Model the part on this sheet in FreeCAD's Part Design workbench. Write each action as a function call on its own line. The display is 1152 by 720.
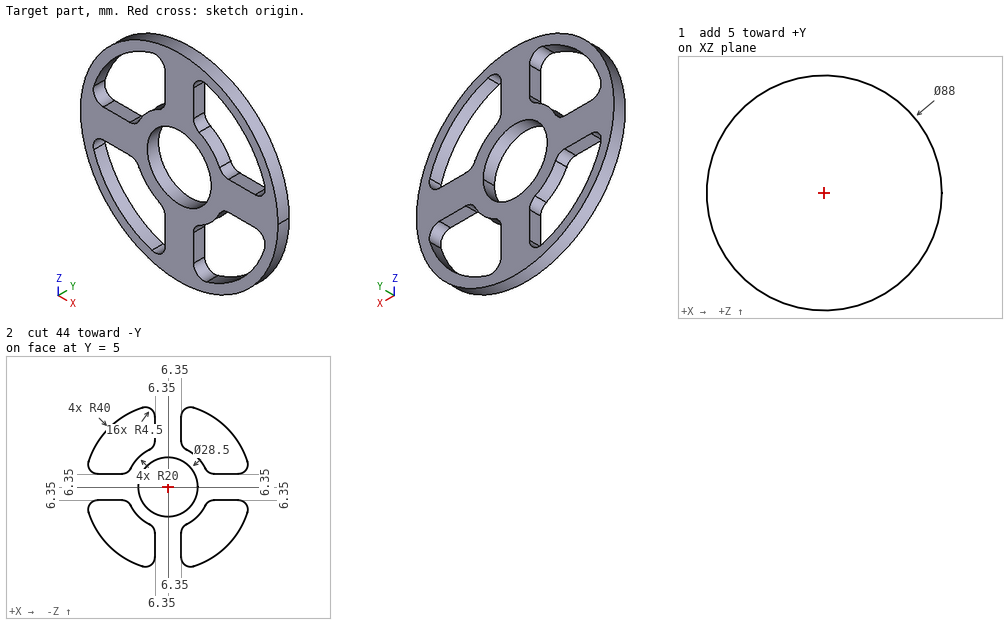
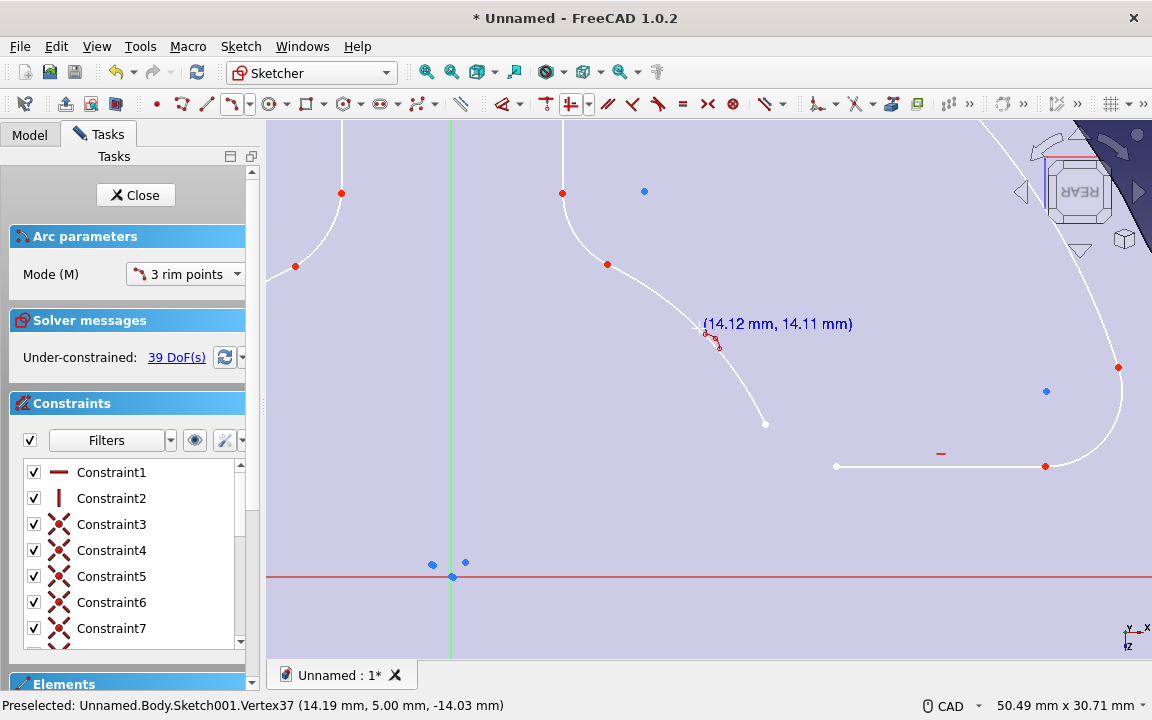
scroll(702, 328, down, 7)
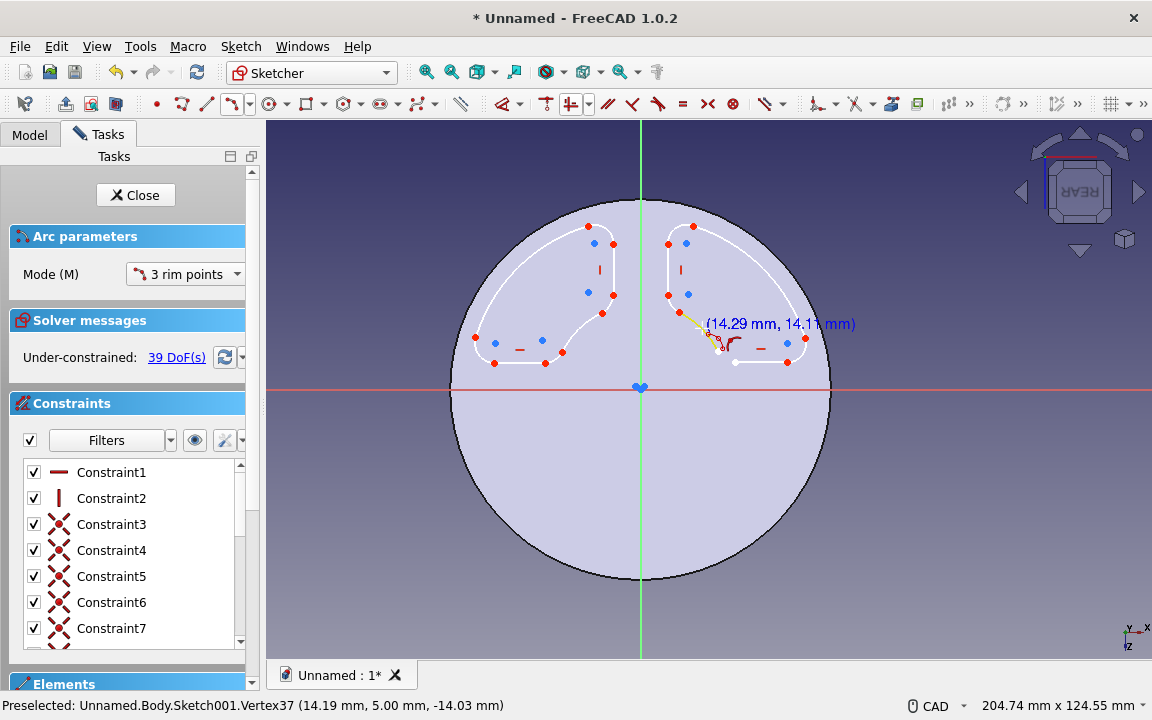
click(718, 352)
click(736, 362)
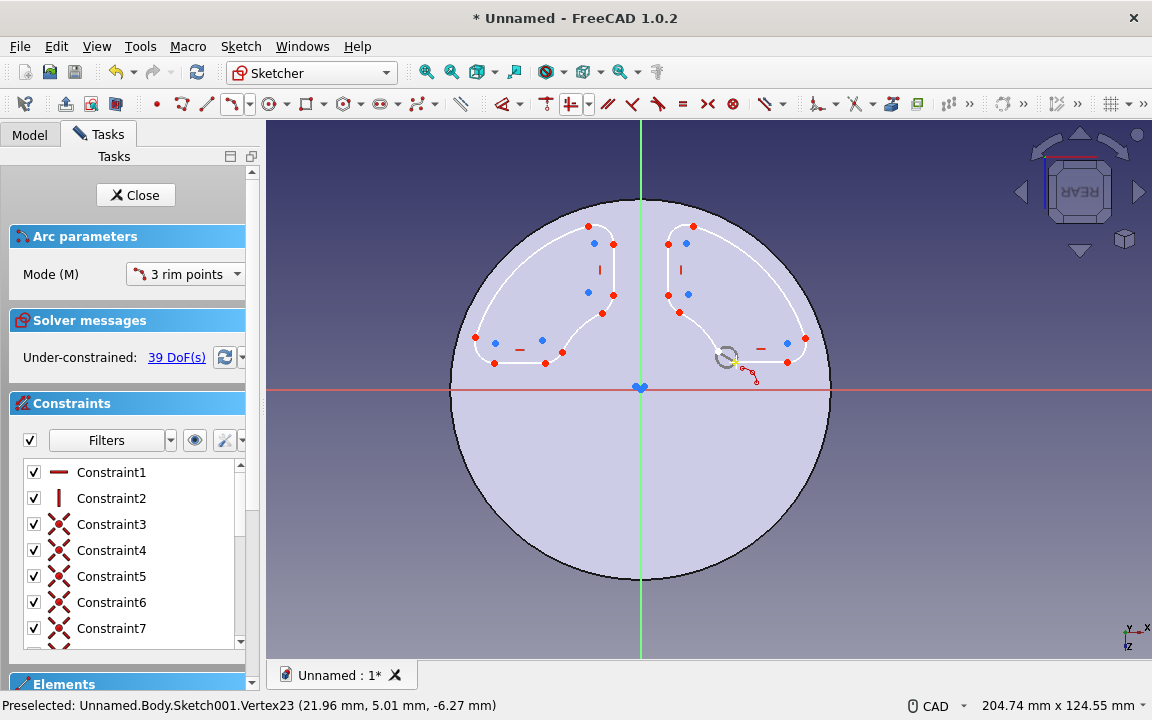
scroll(725, 359, up, 9)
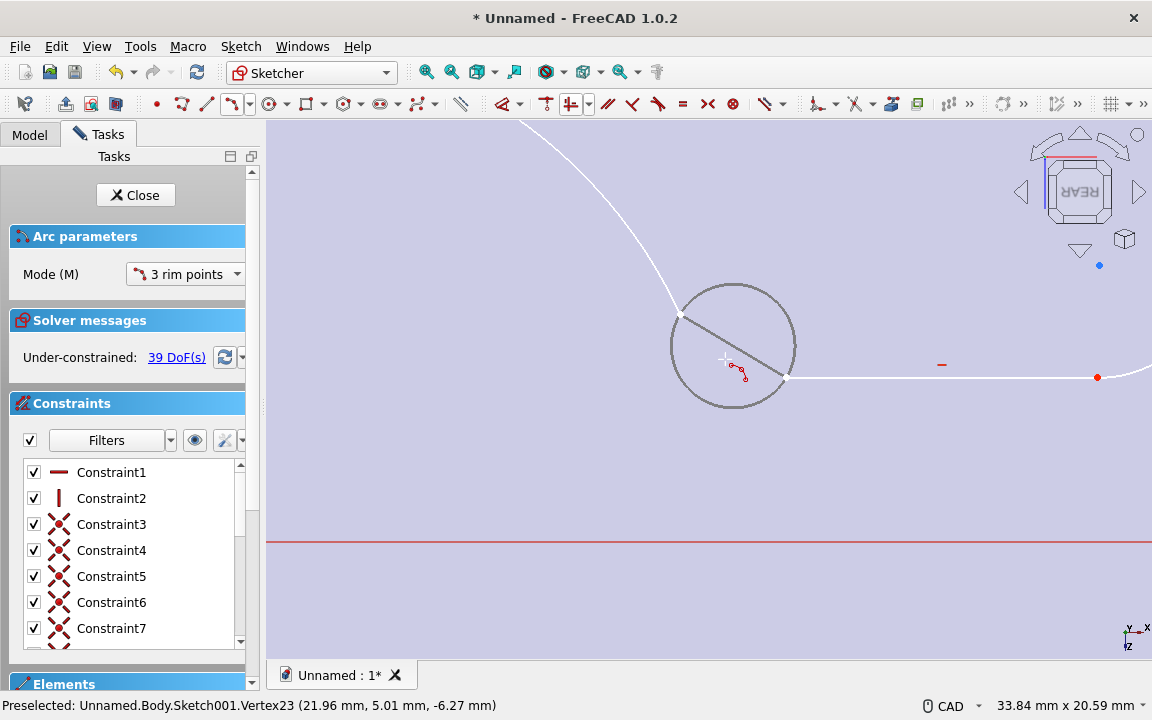
click(724, 358)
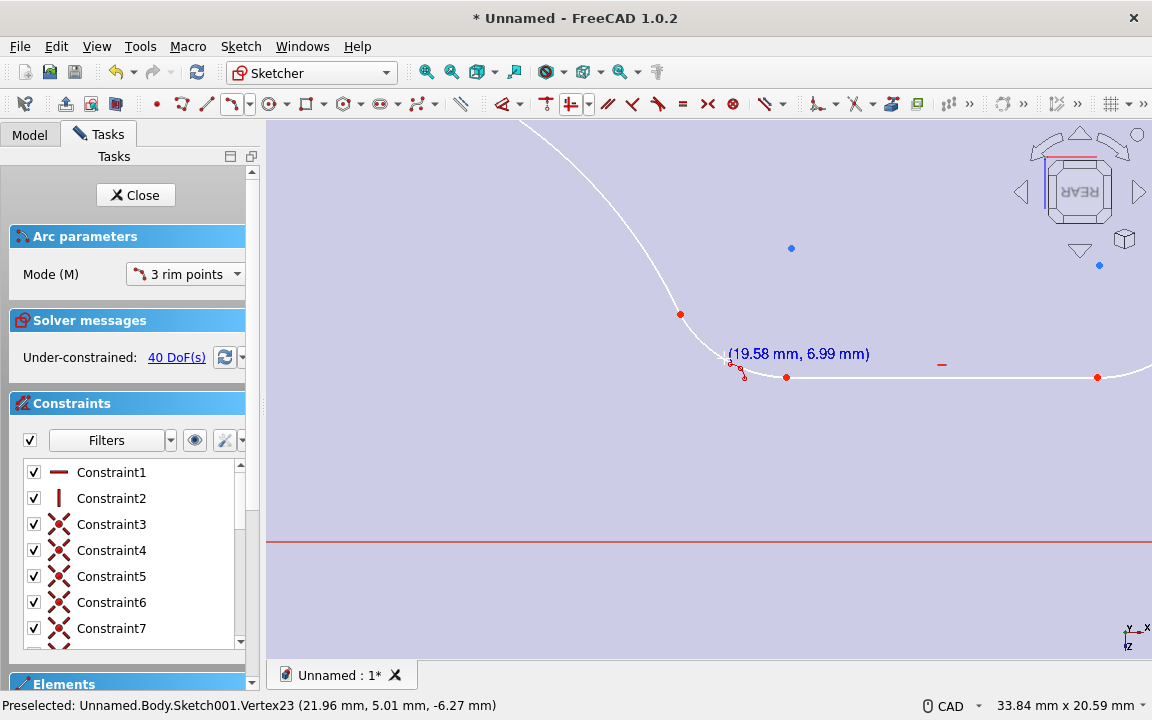
key(g)
key(l)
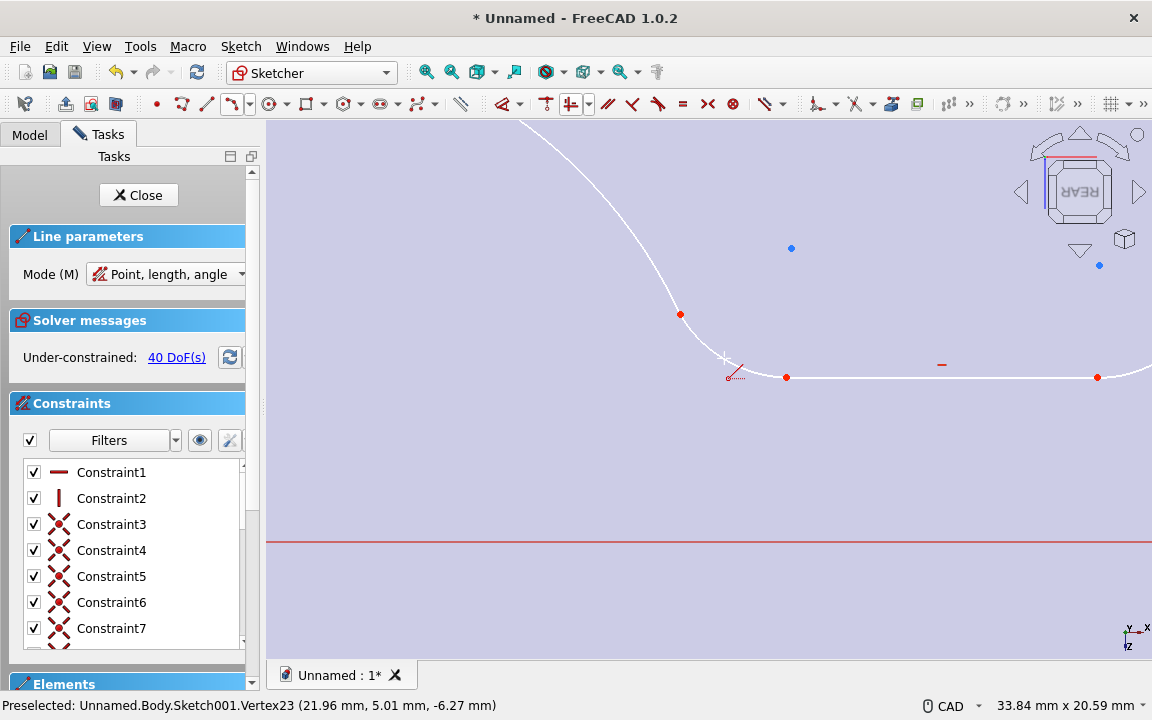
scroll(725, 359, down, 9)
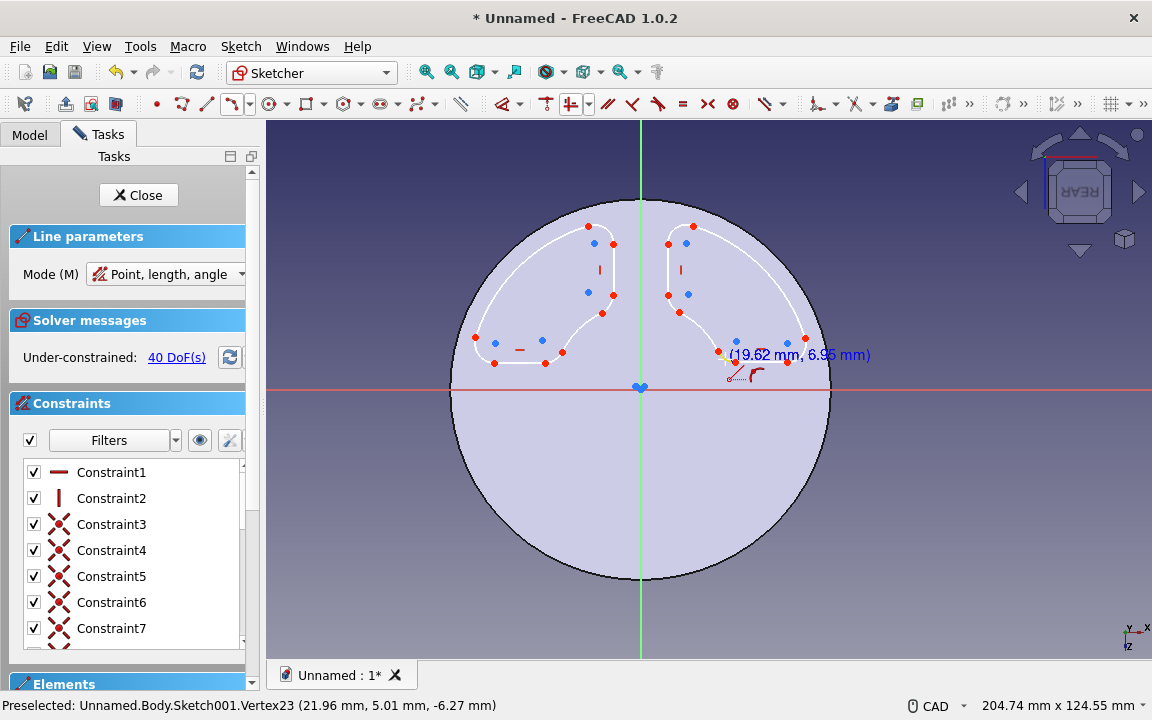
click(787, 417)
click(736, 417)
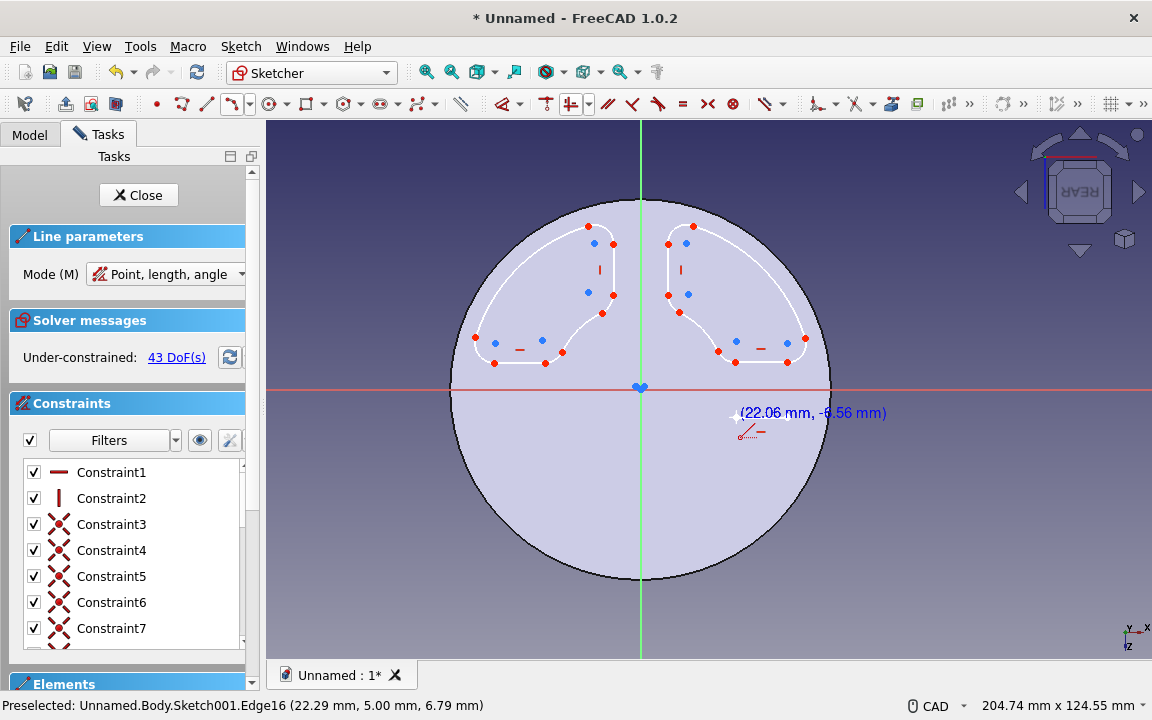
click(668, 485)
click(668, 536)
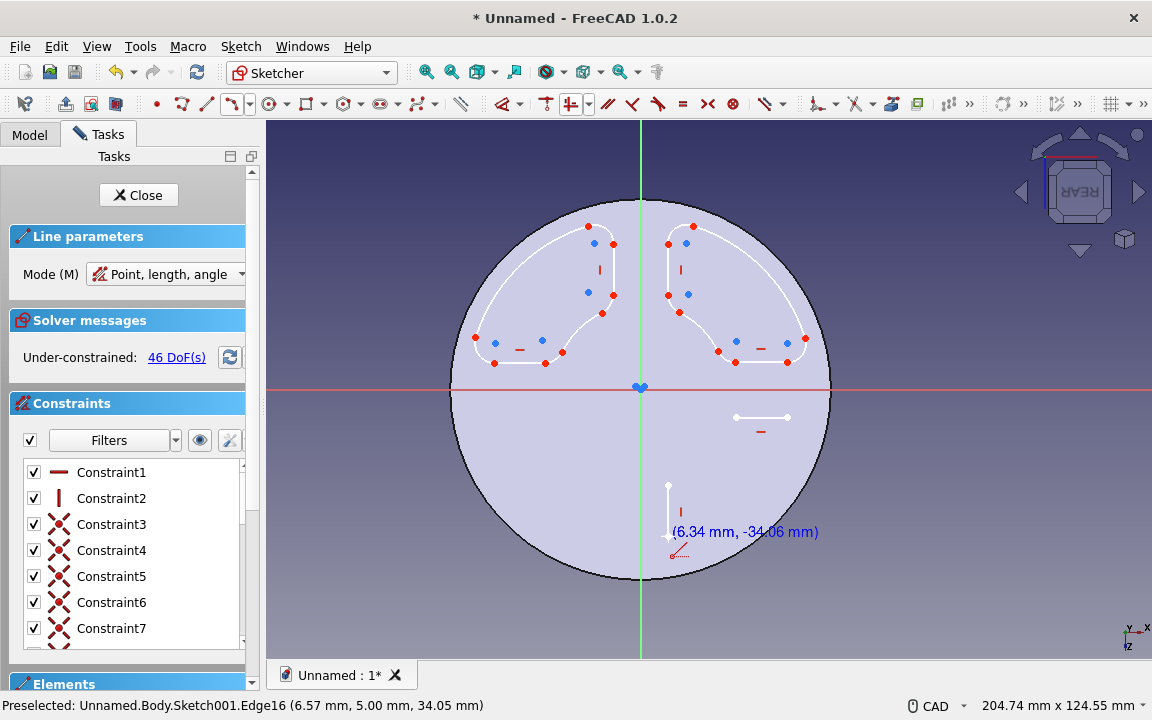
key(g)
key(3)
key(a)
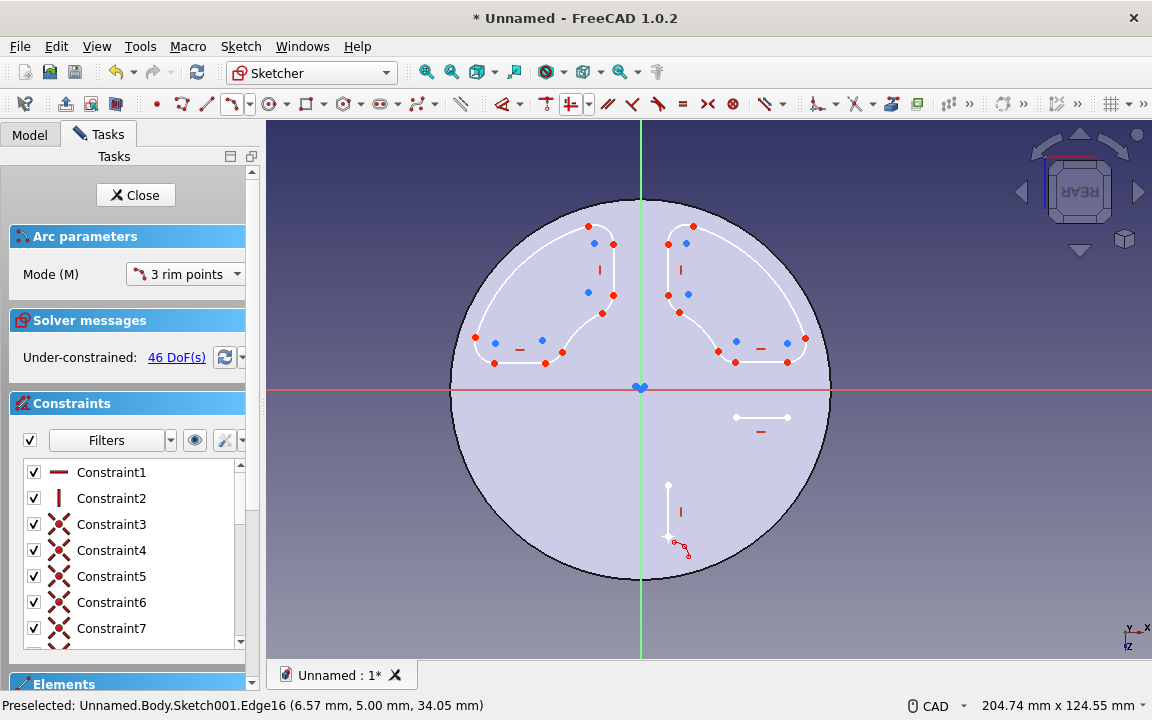
click(736, 418)
click(718, 428)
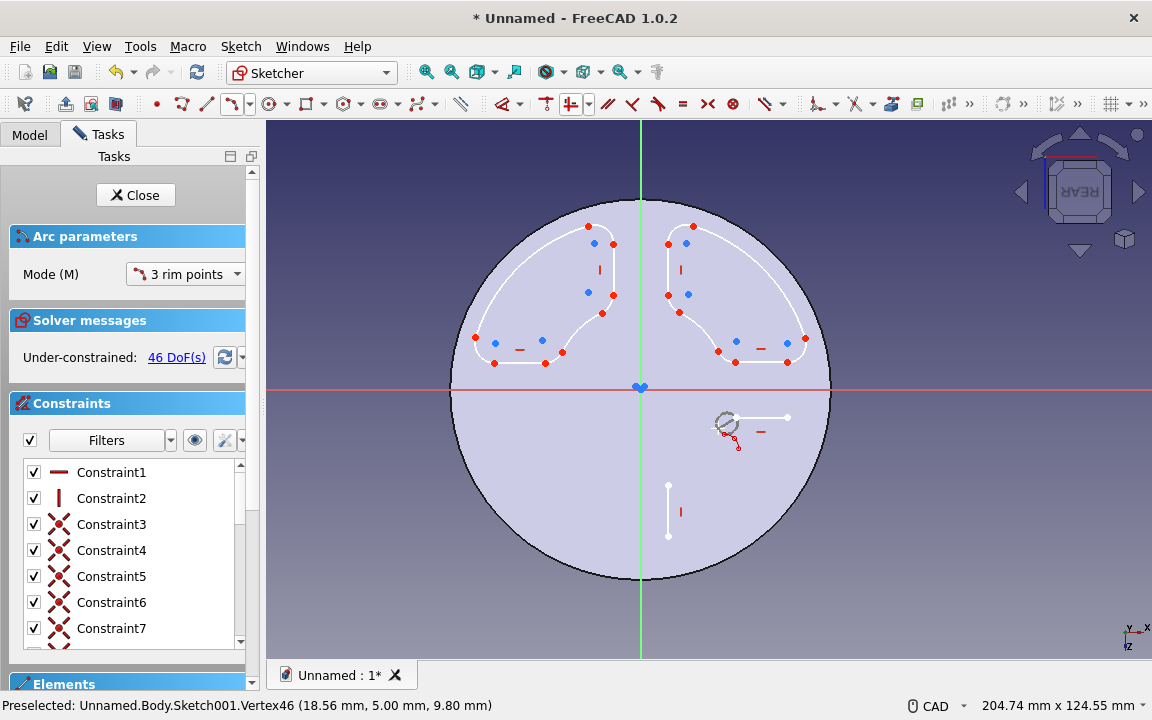
scroll(725, 420, up, 9)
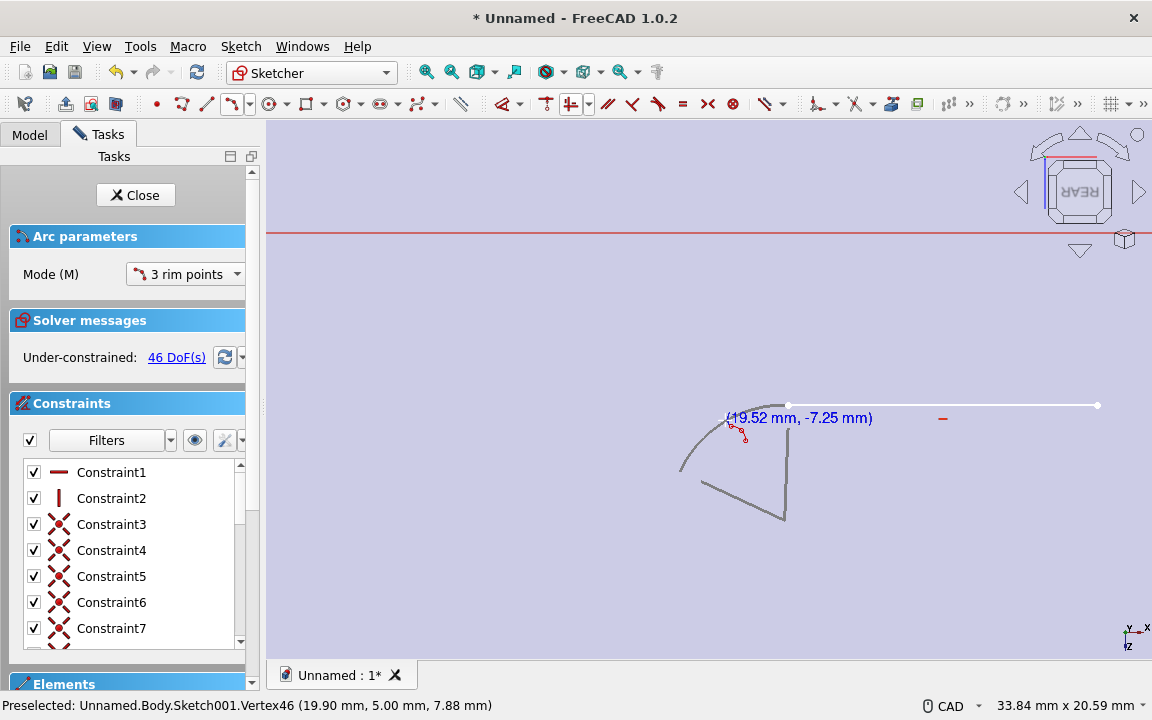
click(724, 417)